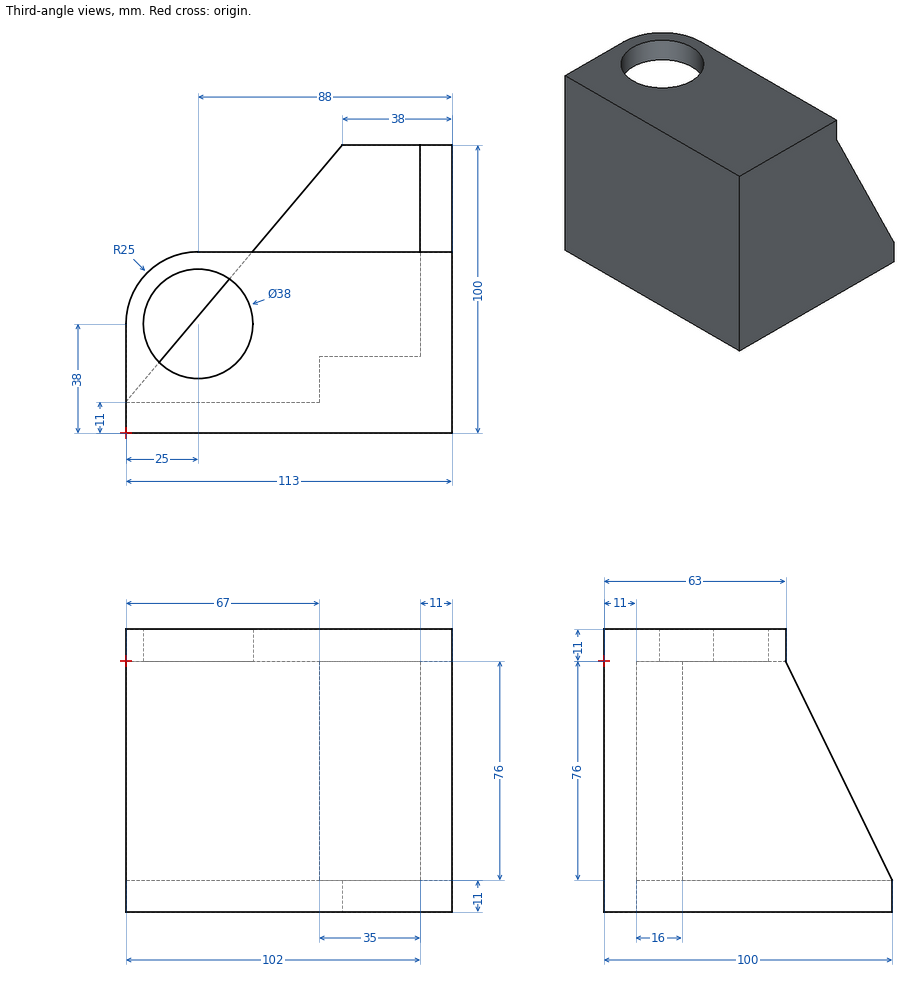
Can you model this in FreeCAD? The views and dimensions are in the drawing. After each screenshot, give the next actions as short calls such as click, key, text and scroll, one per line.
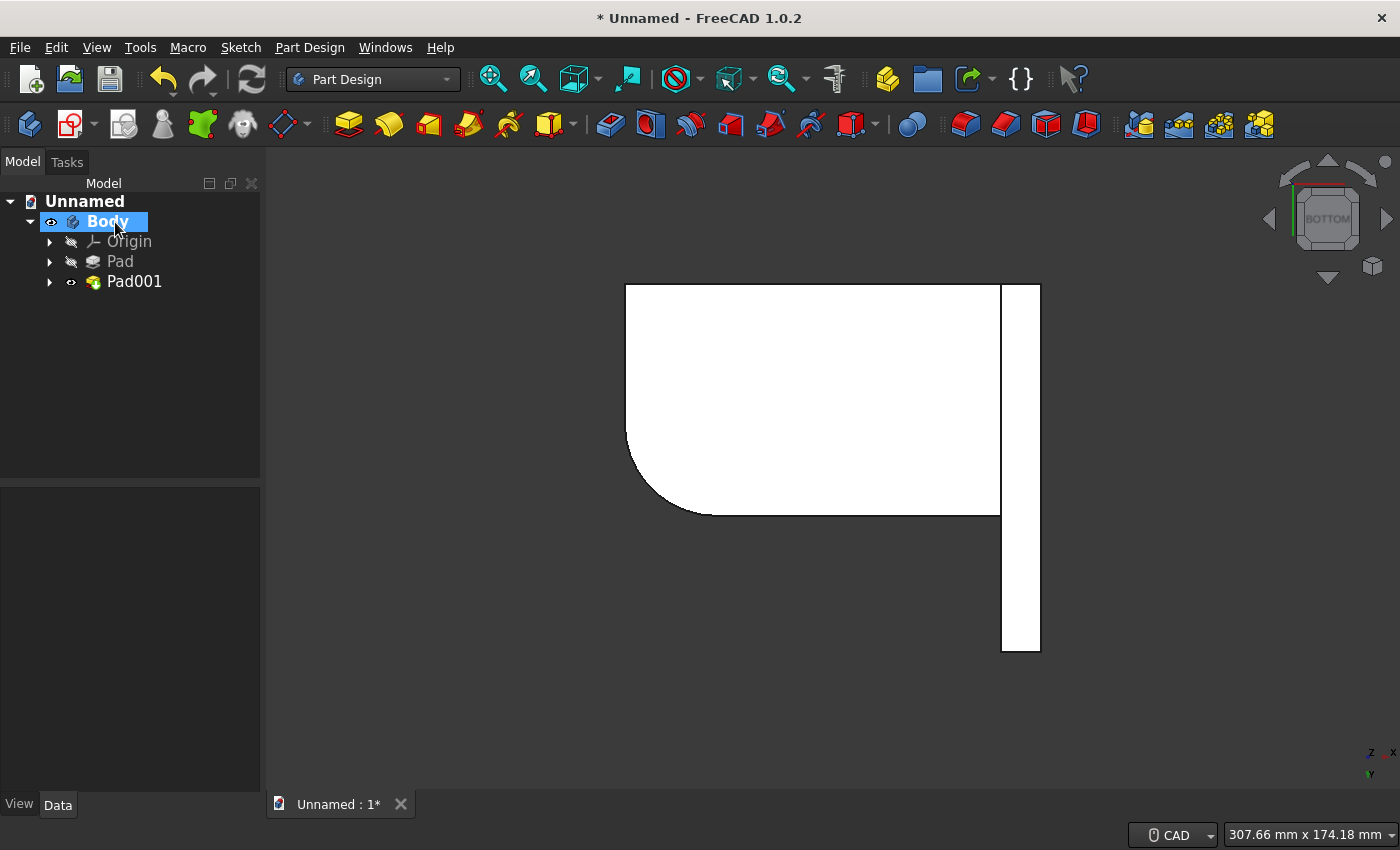
click(1021, 625)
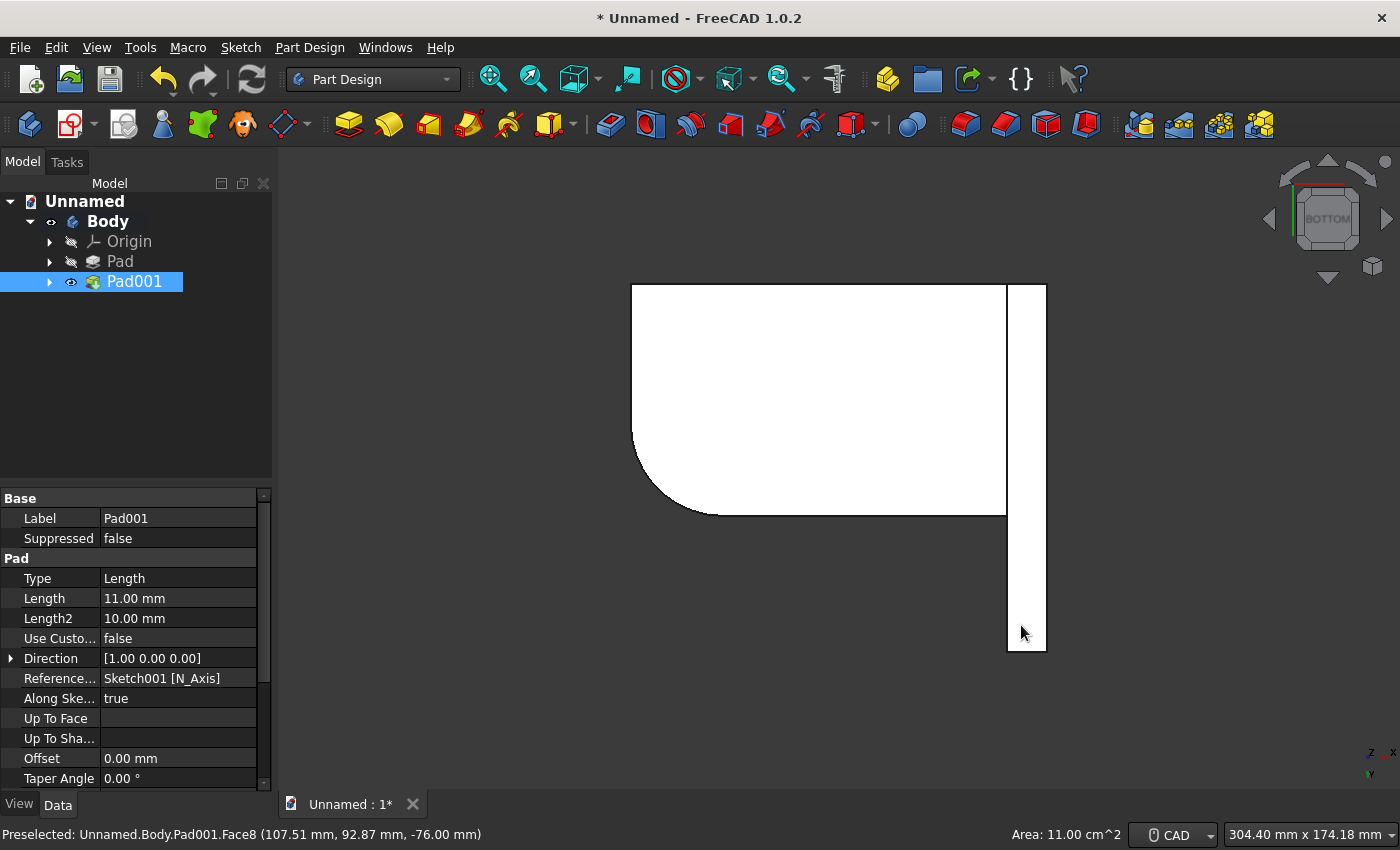
click(70, 124)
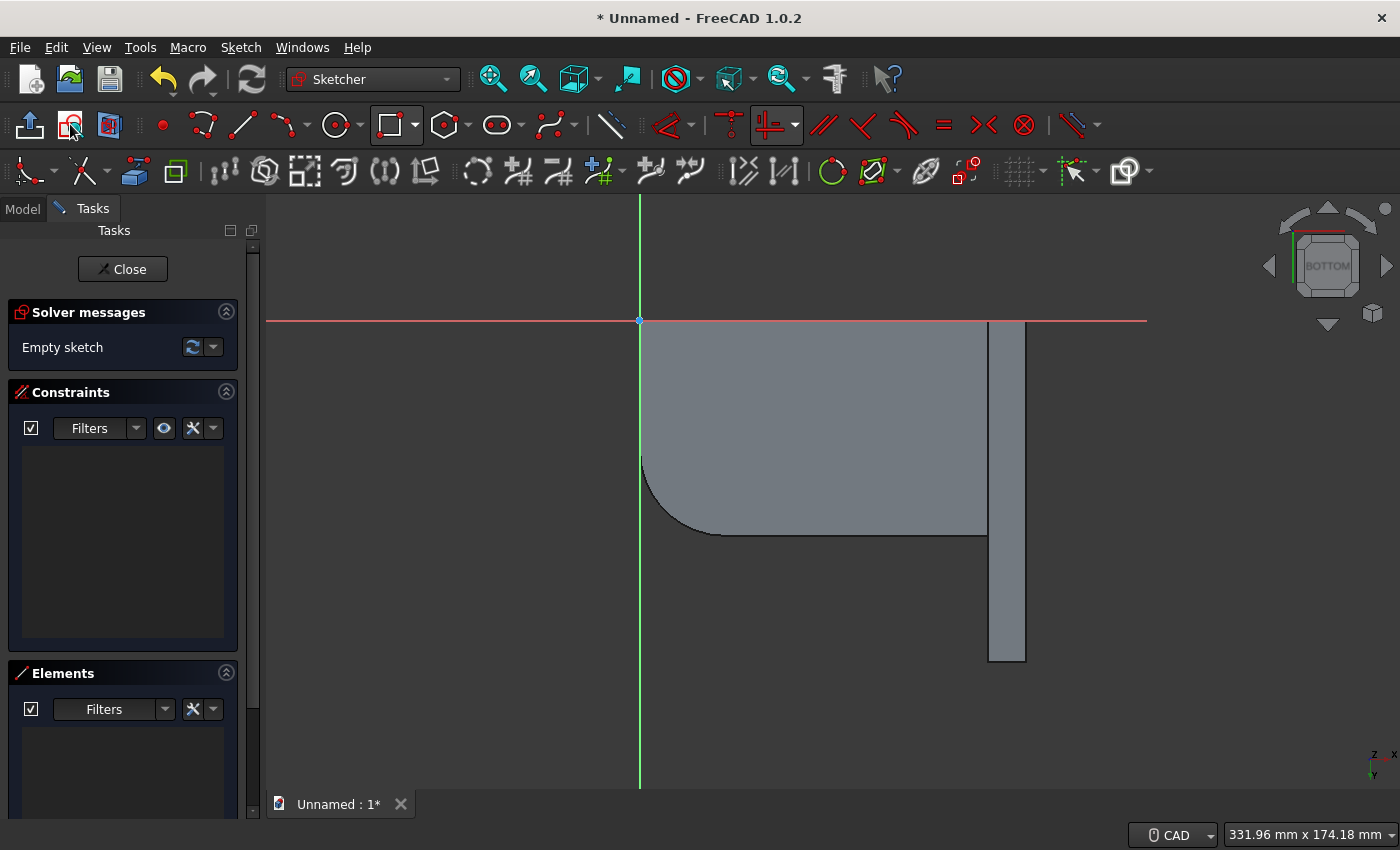
key(g)
key(m)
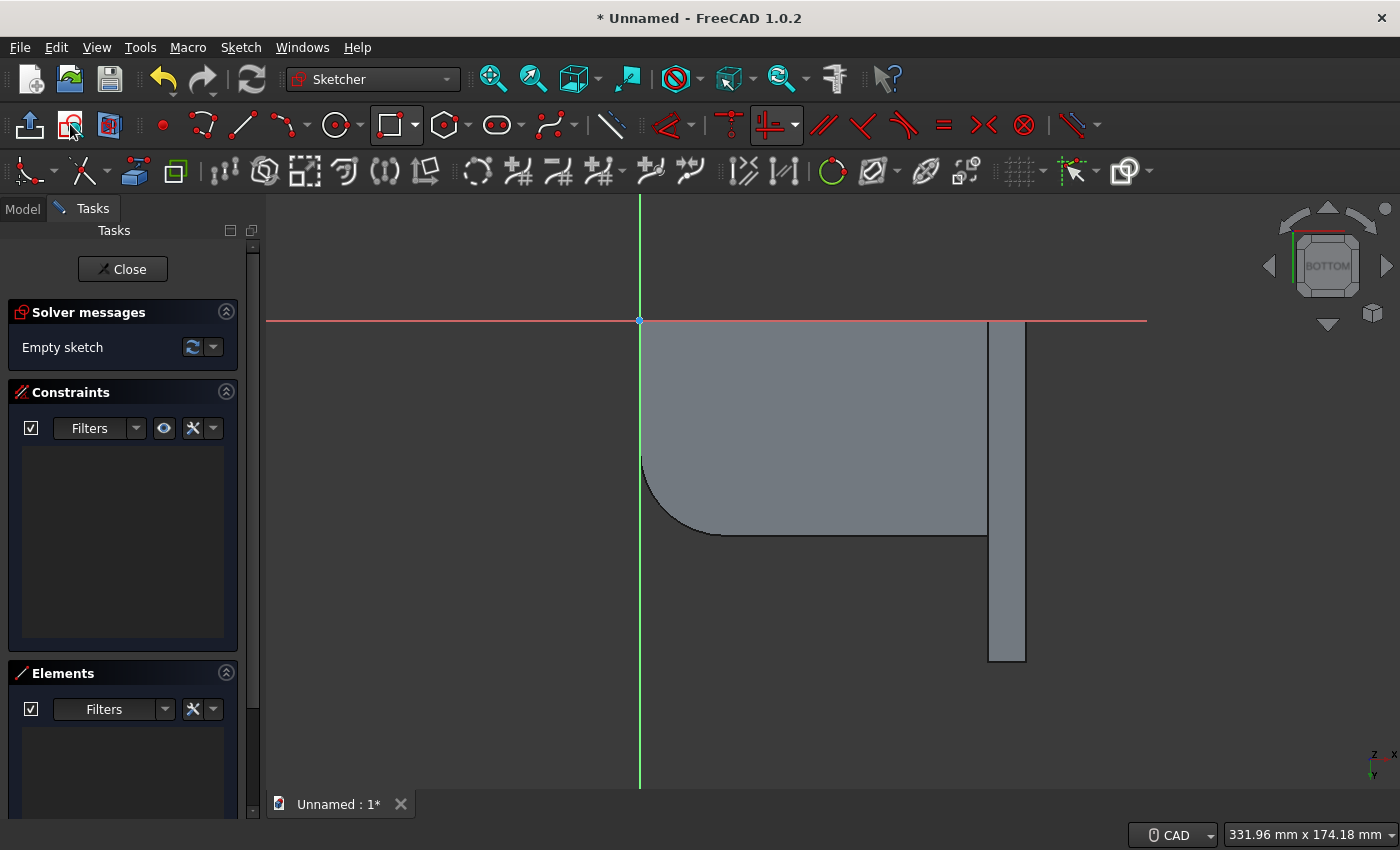
click(640, 321)
click(649, 358)
click(896, 662)
click(1026, 662)
click(1026, 330)
click(640, 321)
key(Escape)
key(Escape)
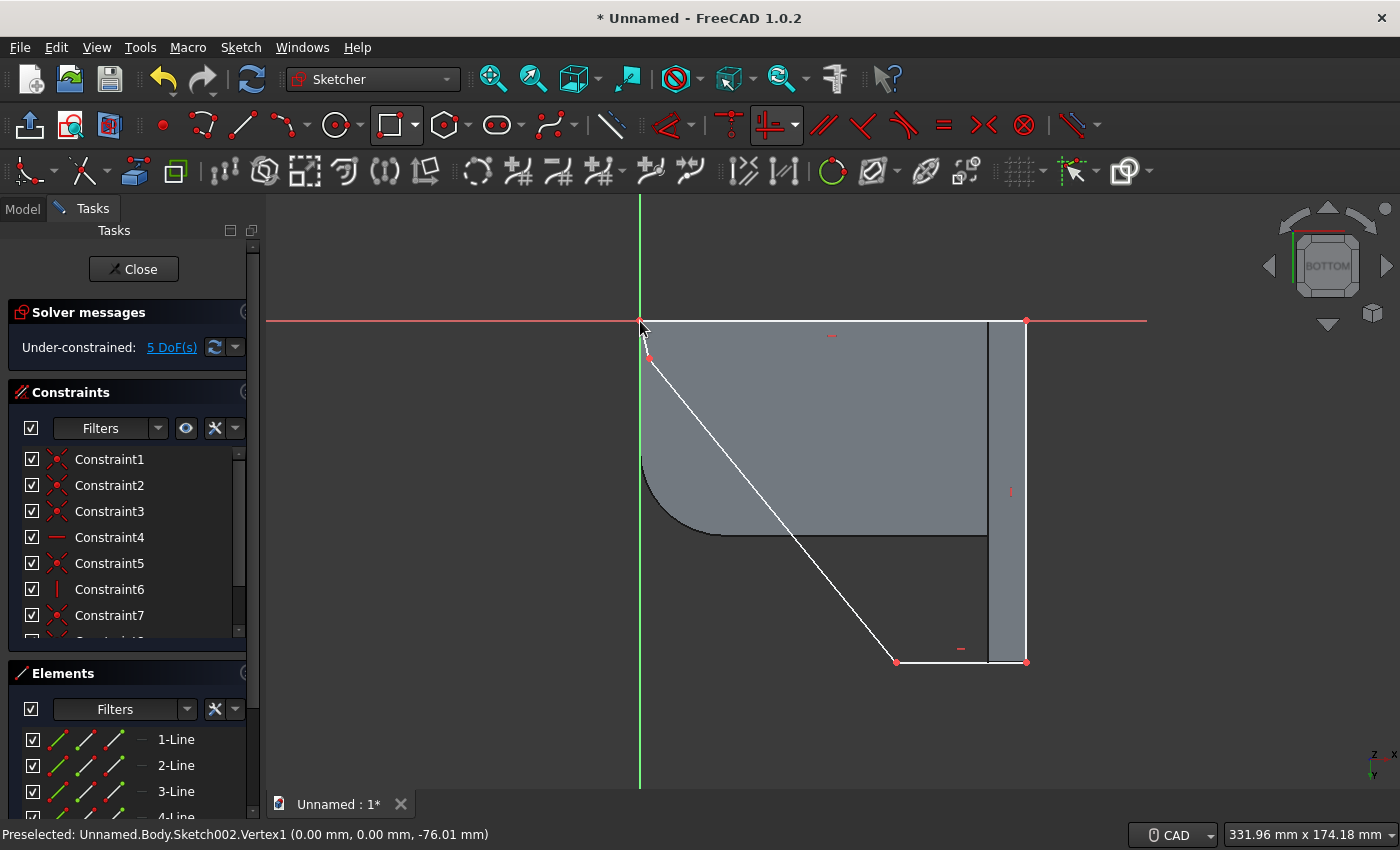
click(643, 332)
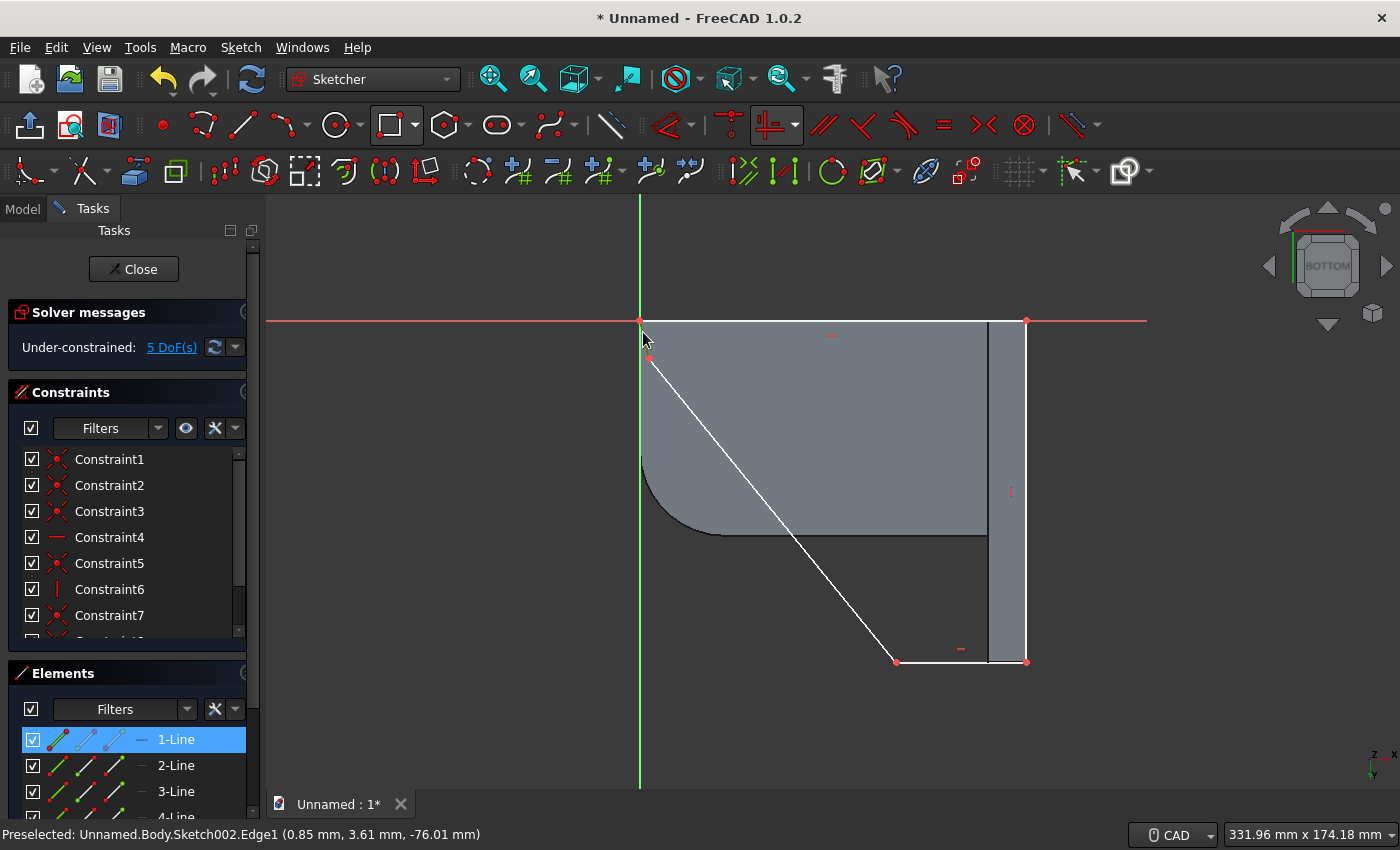
key(v)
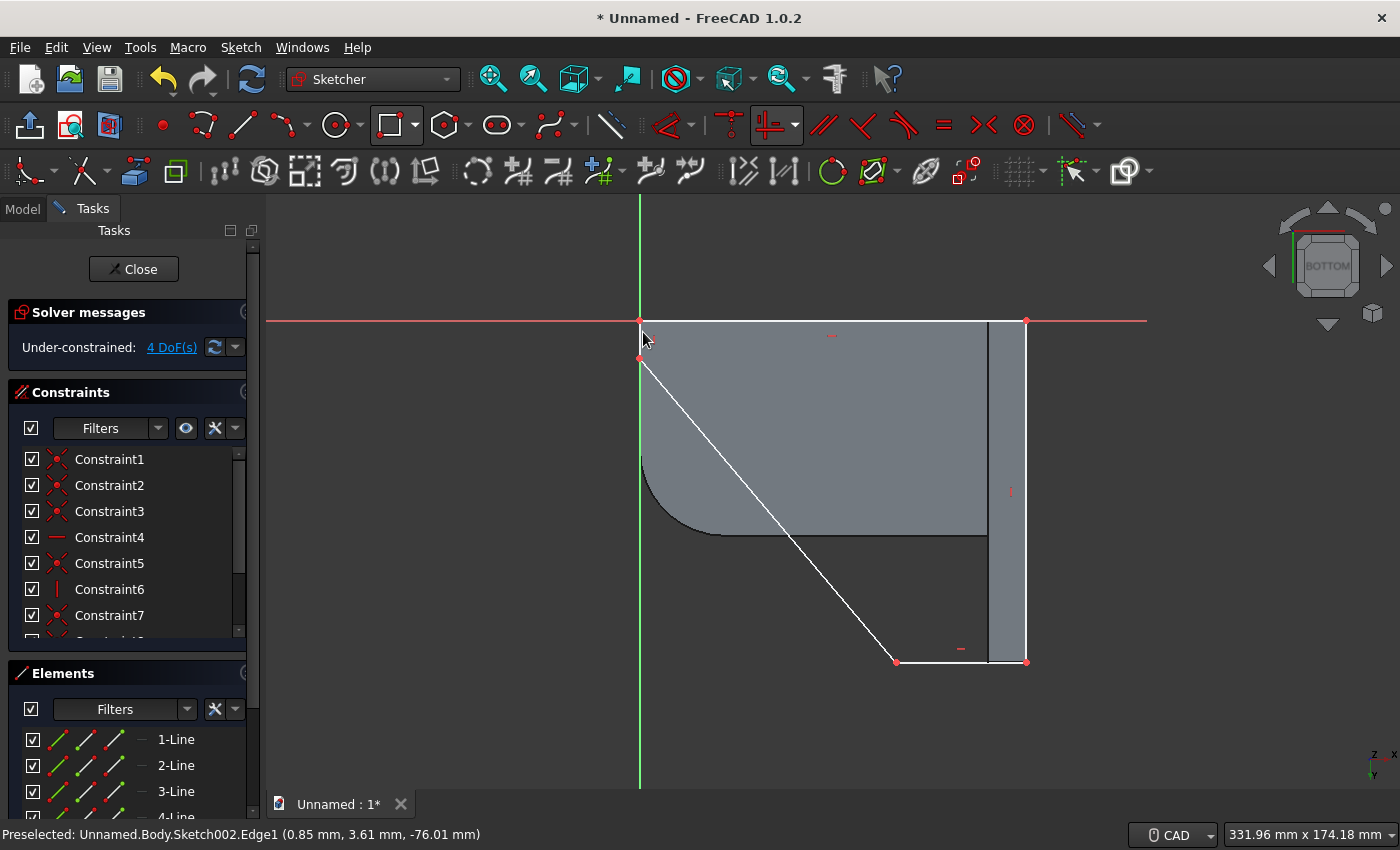
click(666, 126)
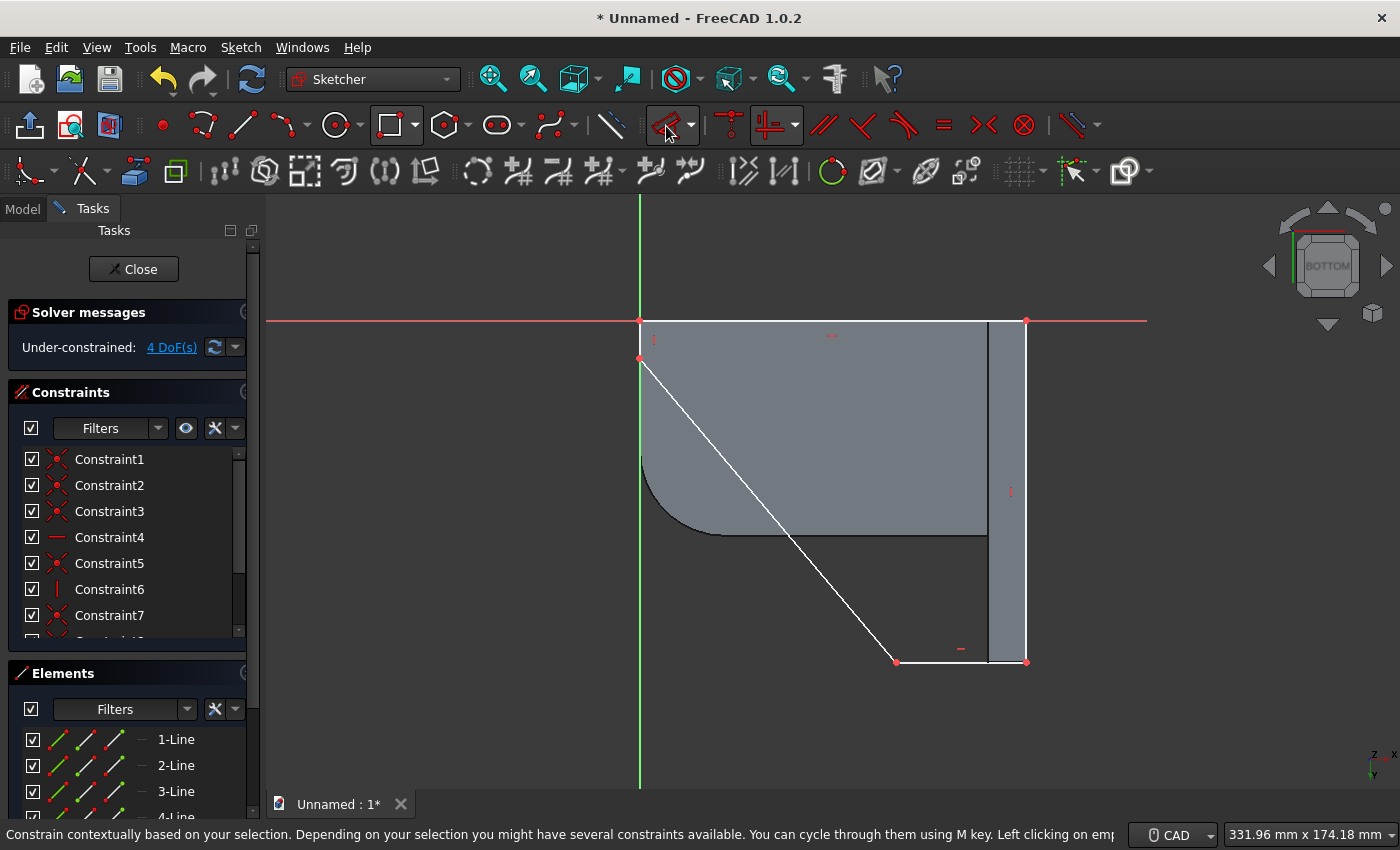
click(640, 332)
click(606, 340)